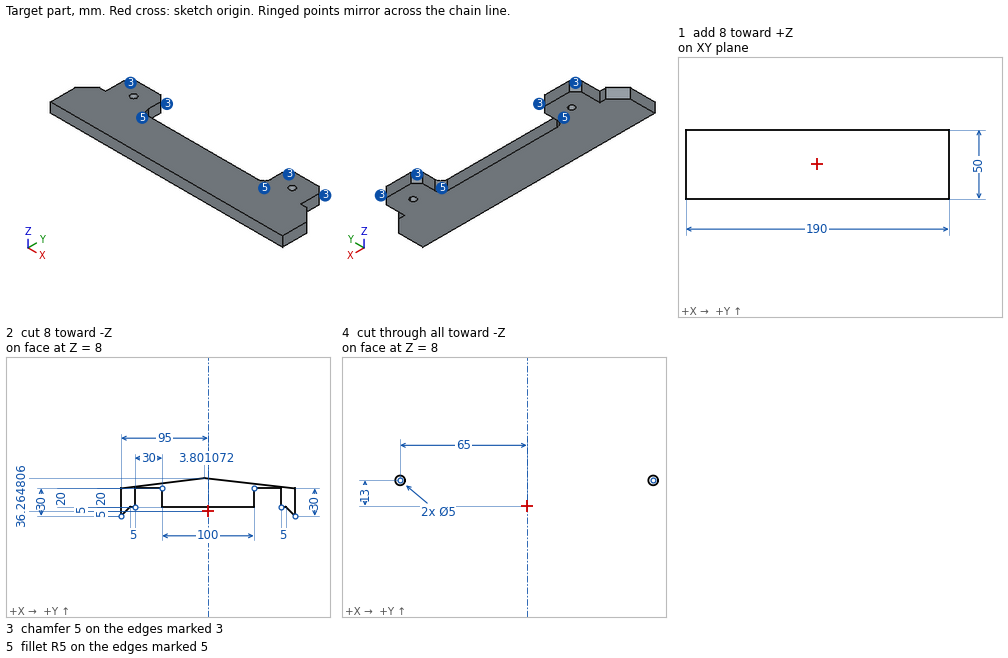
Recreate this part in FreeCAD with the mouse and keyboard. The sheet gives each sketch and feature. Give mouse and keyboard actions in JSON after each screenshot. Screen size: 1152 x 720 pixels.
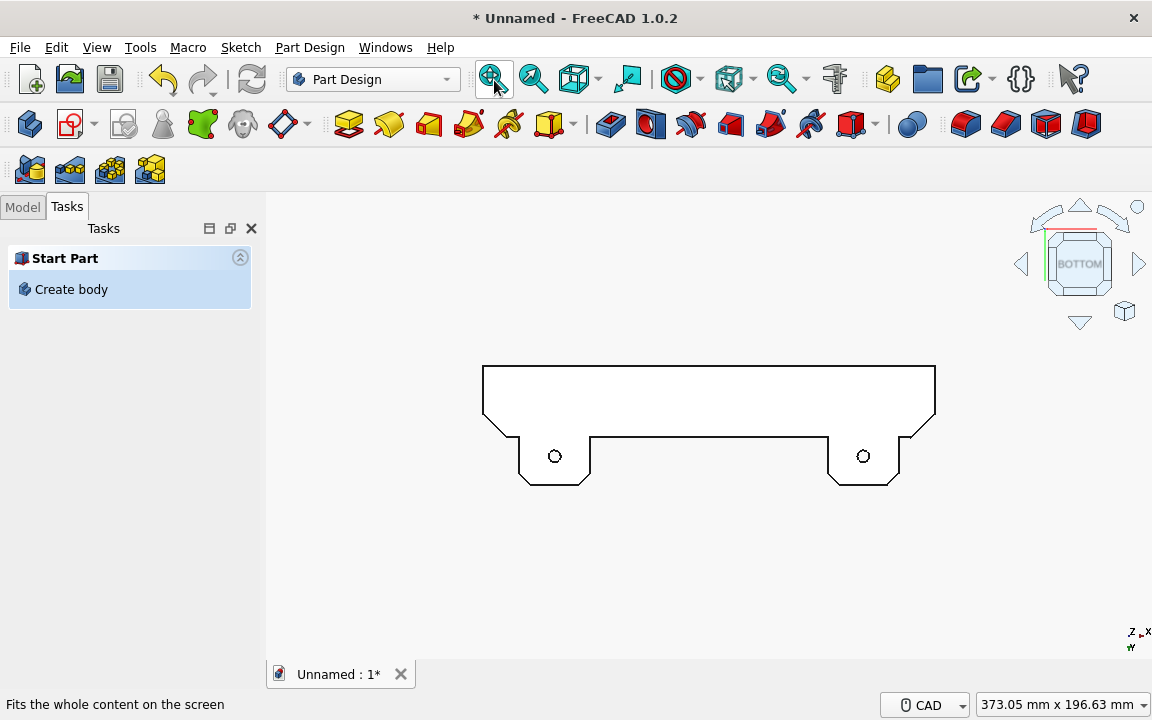
{"action": "key", "text": "4"}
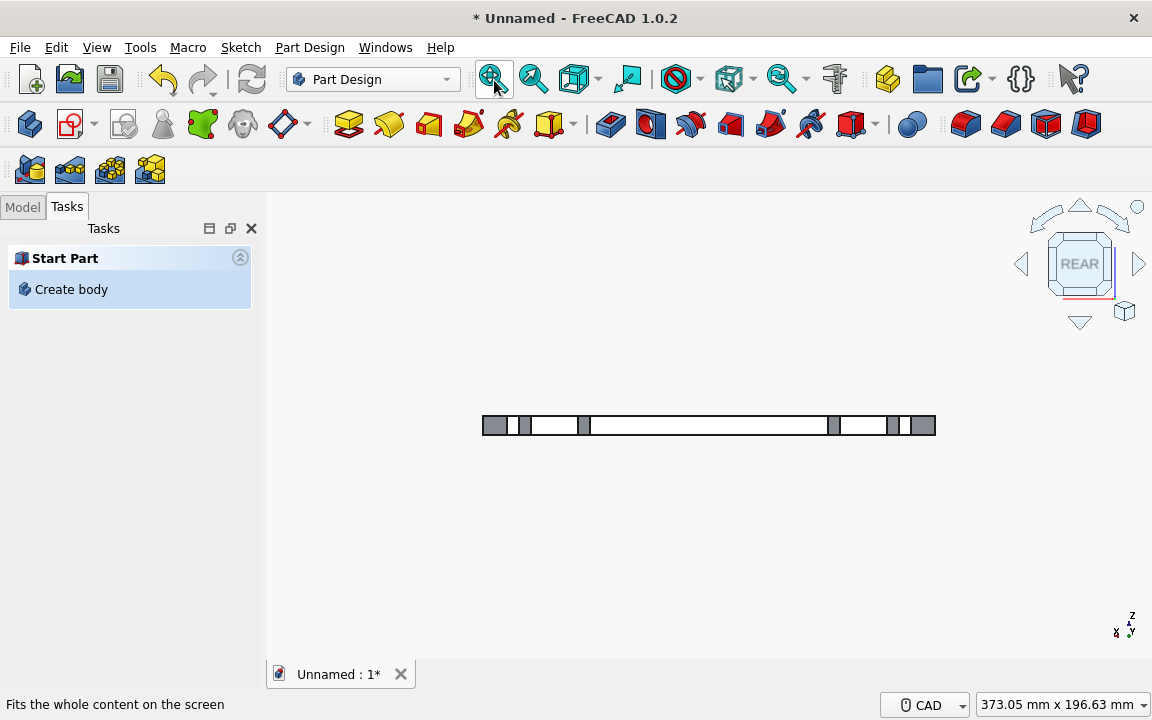
{"action": "scroll", "coordinate": [590, 424], "scroll_direction": "up", "scroll_amount": 4}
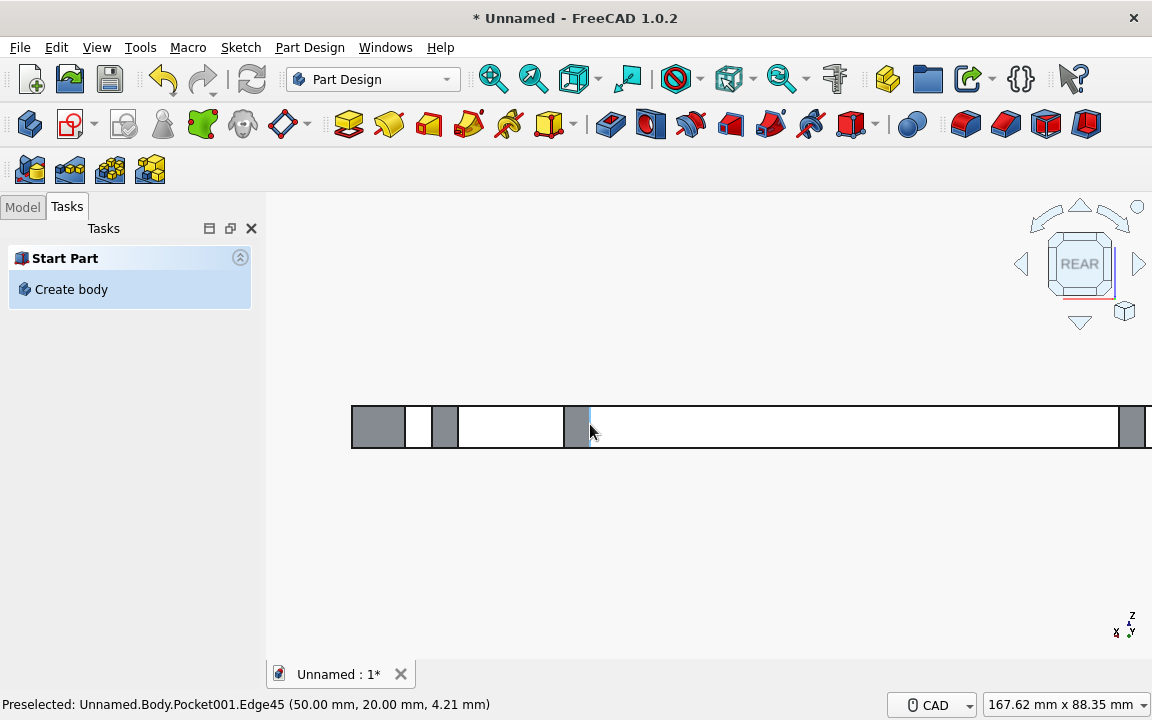
{"action": "left_click", "coordinate": [494, 80]}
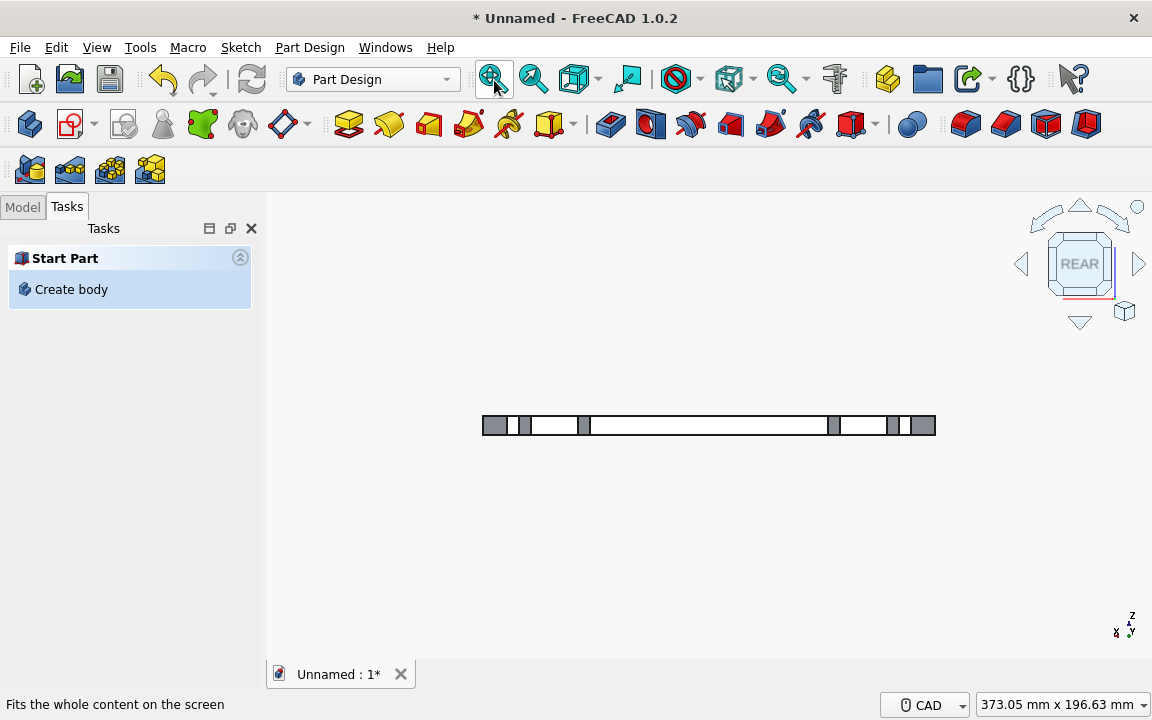
{"action": "key", "text": "6"}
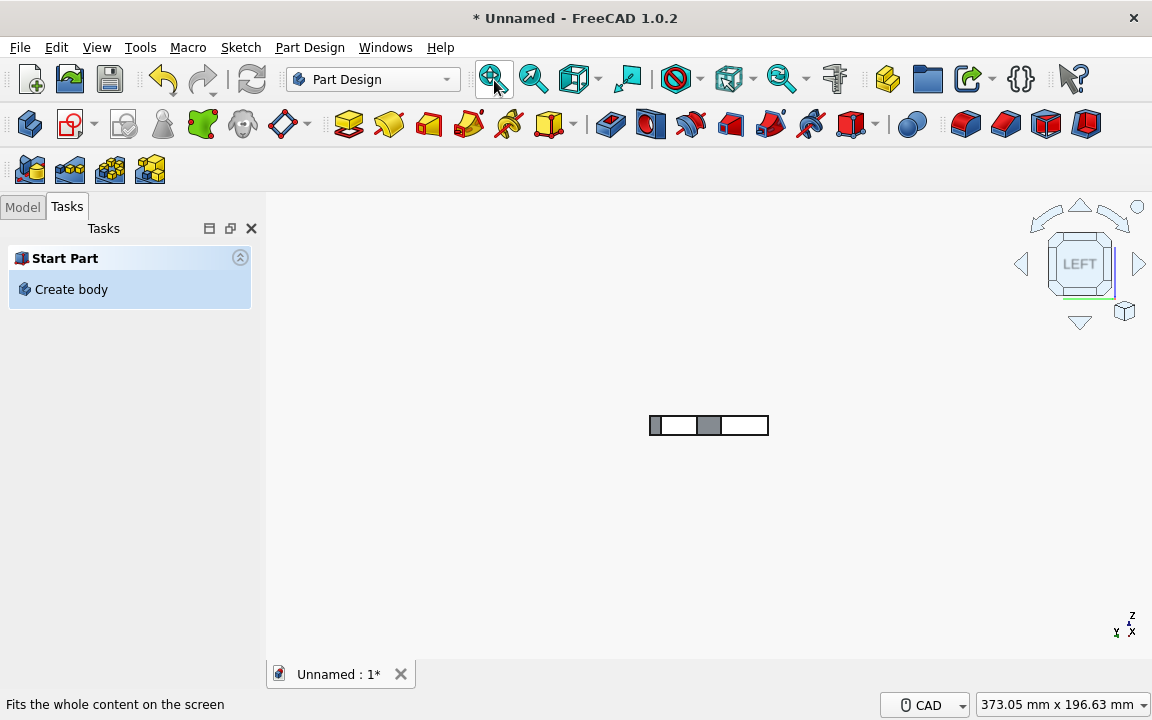
{"action": "left_click", "coordinate": [494, 80]}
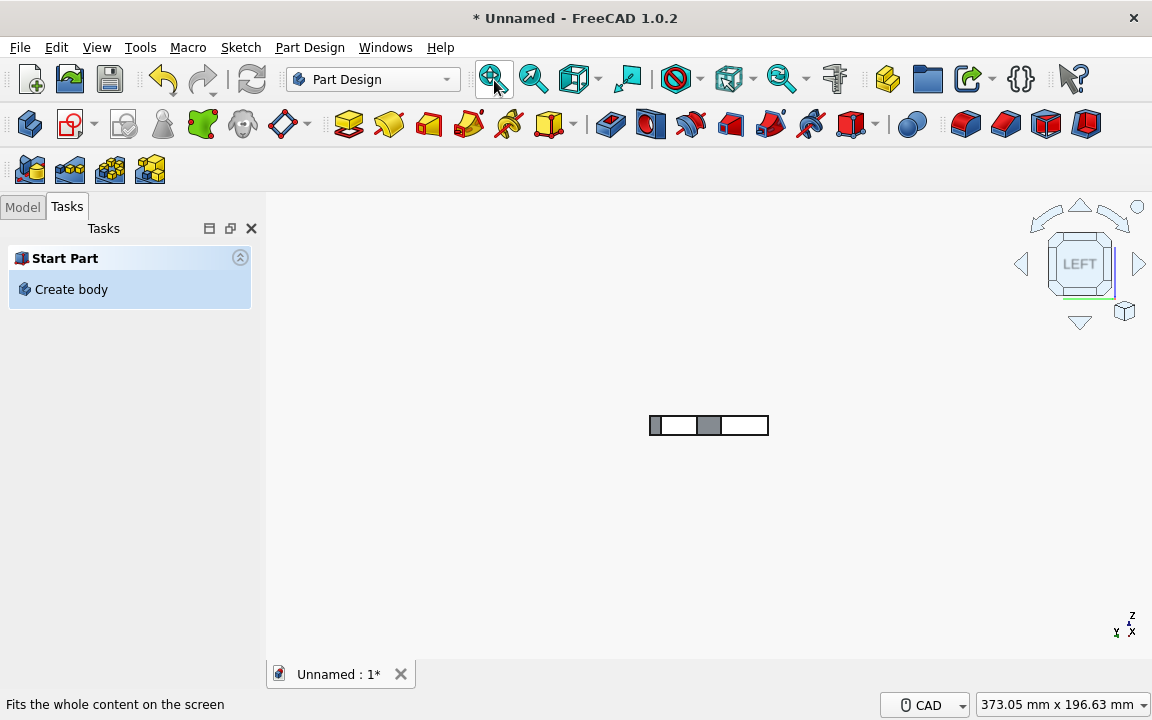
{"action": "scroll", "coordinate": [697, 424], "scroll_direction": "up", "scroll_amount": 4}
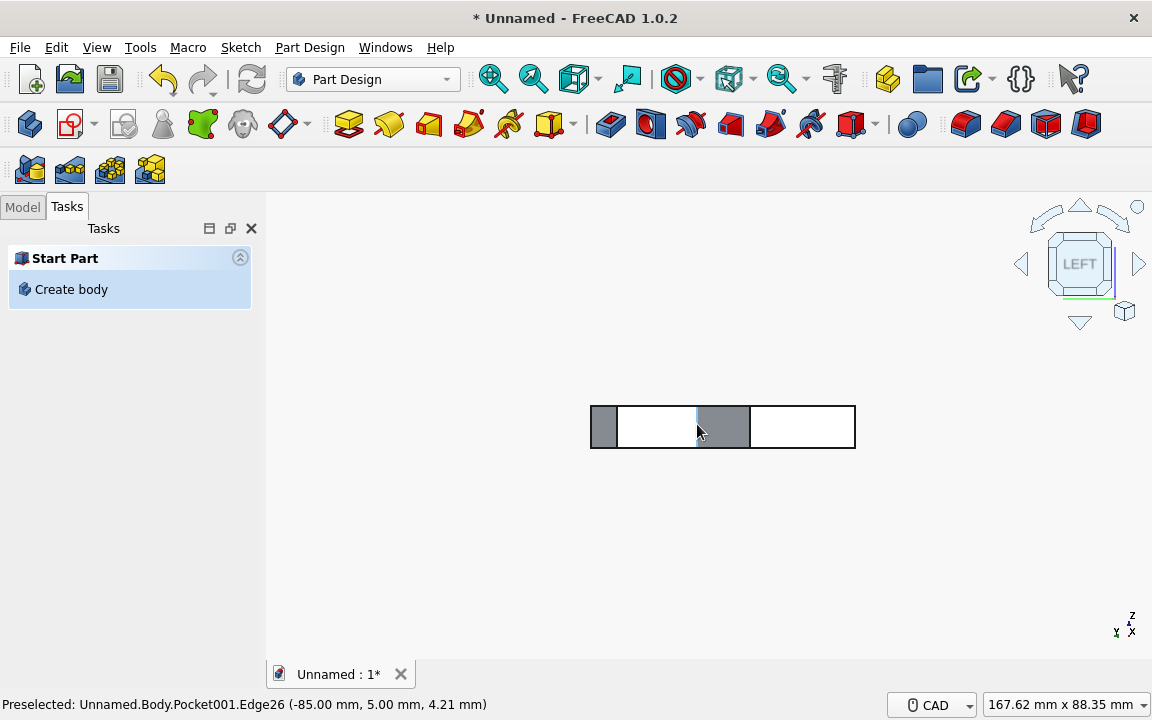
{"action": "left_click", "coordinate": [494, 80]}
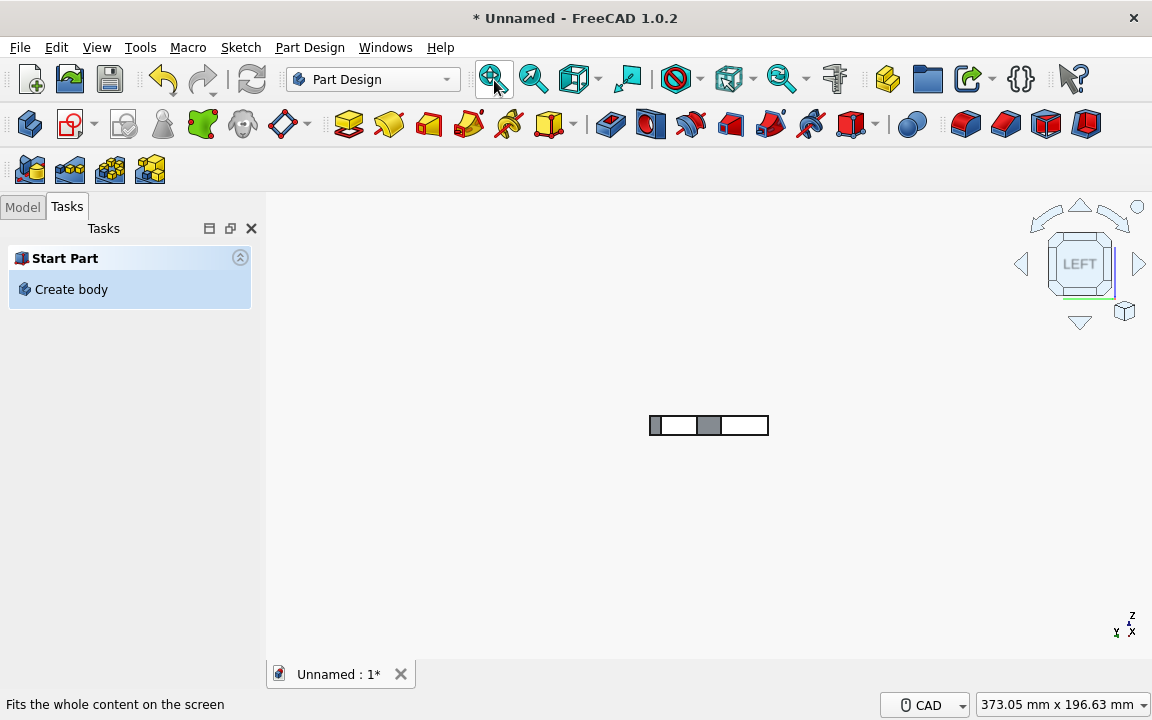
{"action": "key", "text": "v 3"}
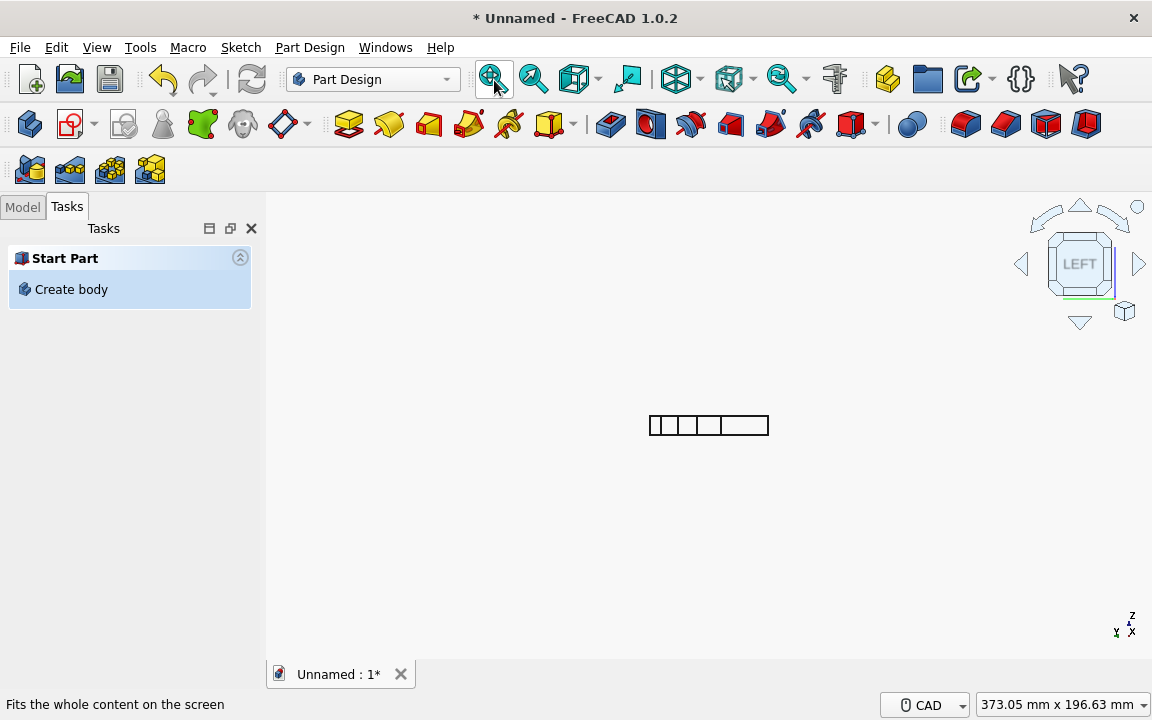
{"action": "key", "text": "0"}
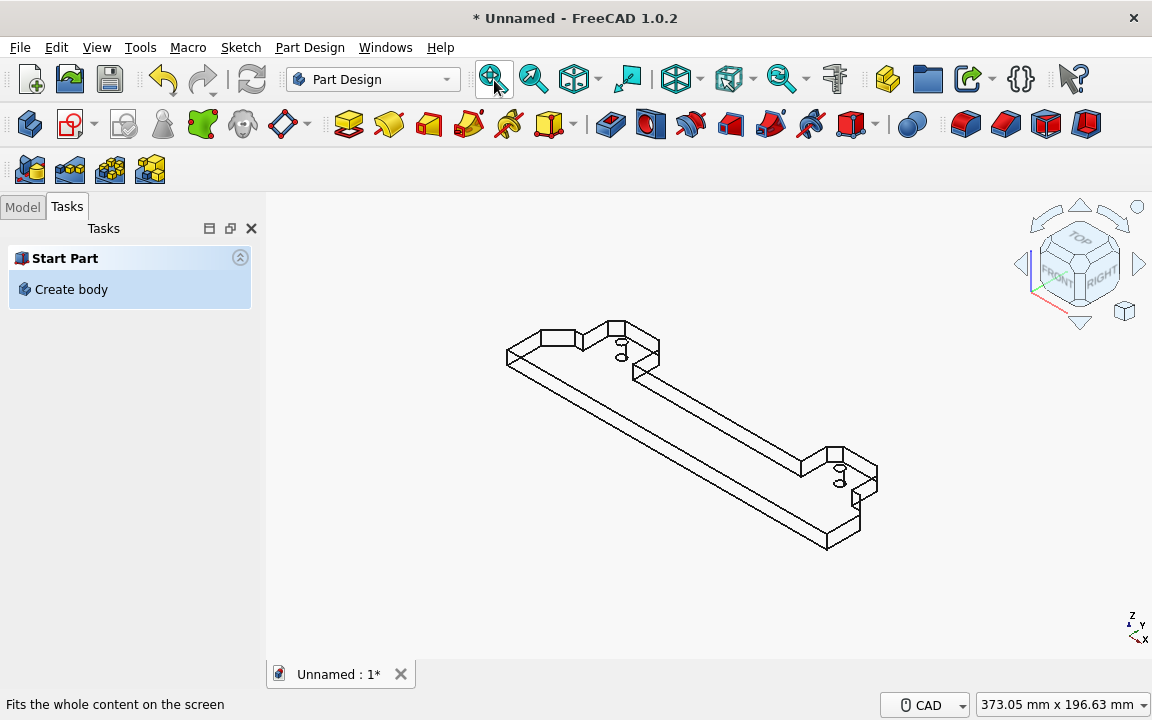
{"action": "left_click", "coordinate": [801, 468]}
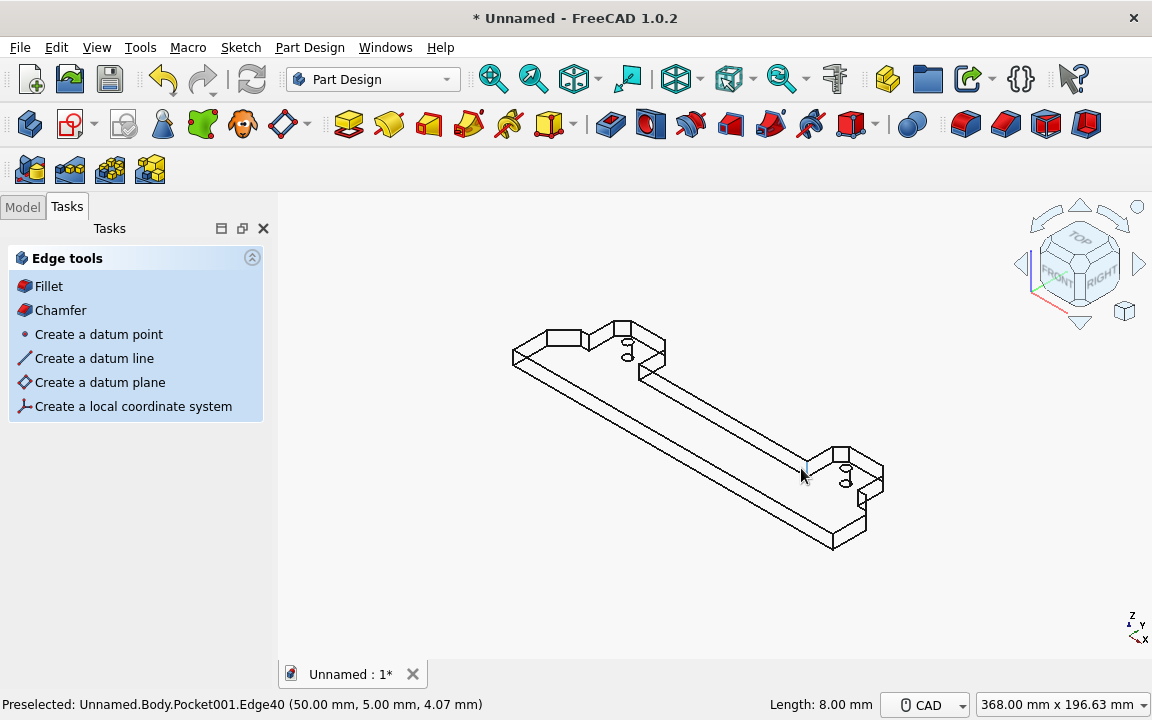
{"action": "left_click", "coordinate": [639, 371], "text": "ctrl"}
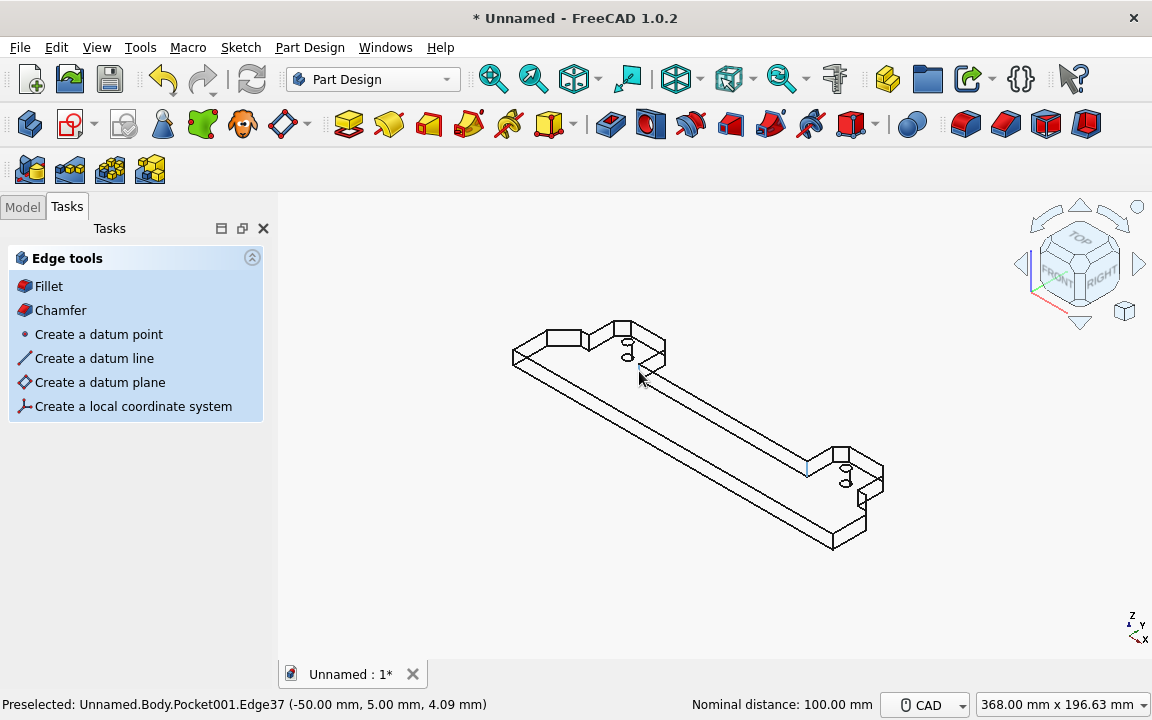
{"action": "key", "text": "v 1"}